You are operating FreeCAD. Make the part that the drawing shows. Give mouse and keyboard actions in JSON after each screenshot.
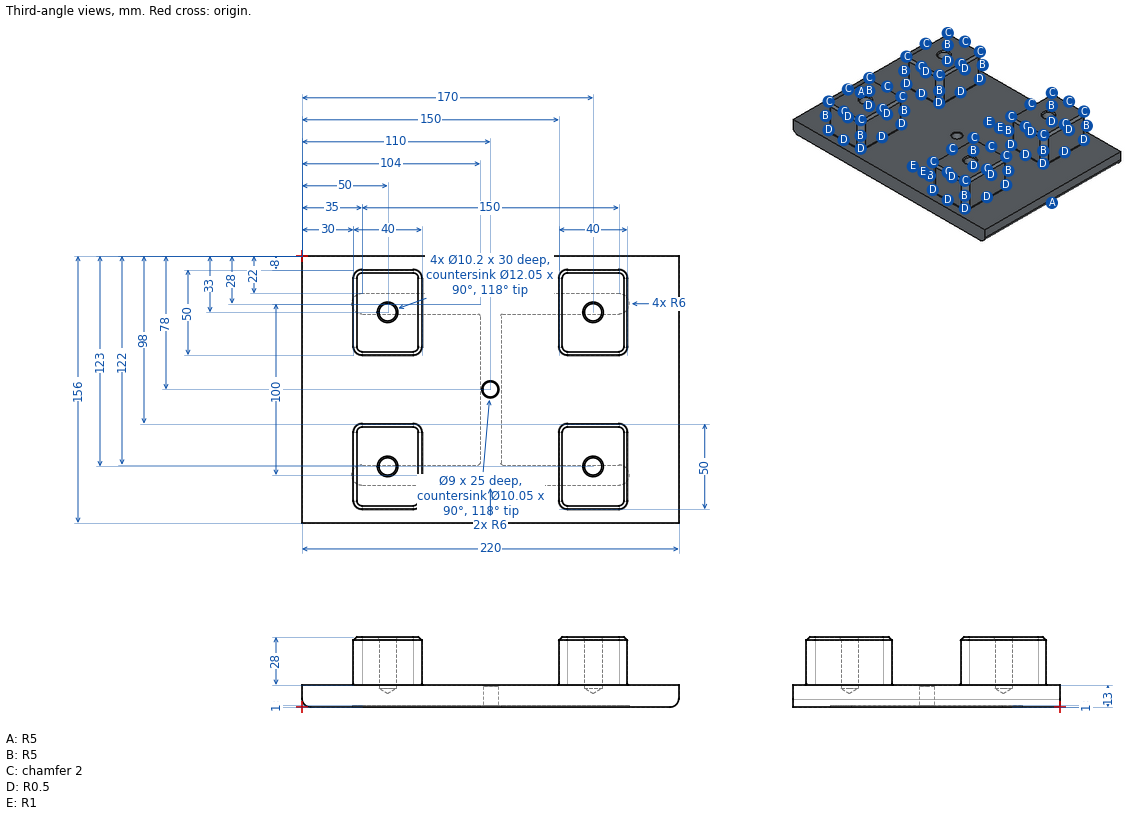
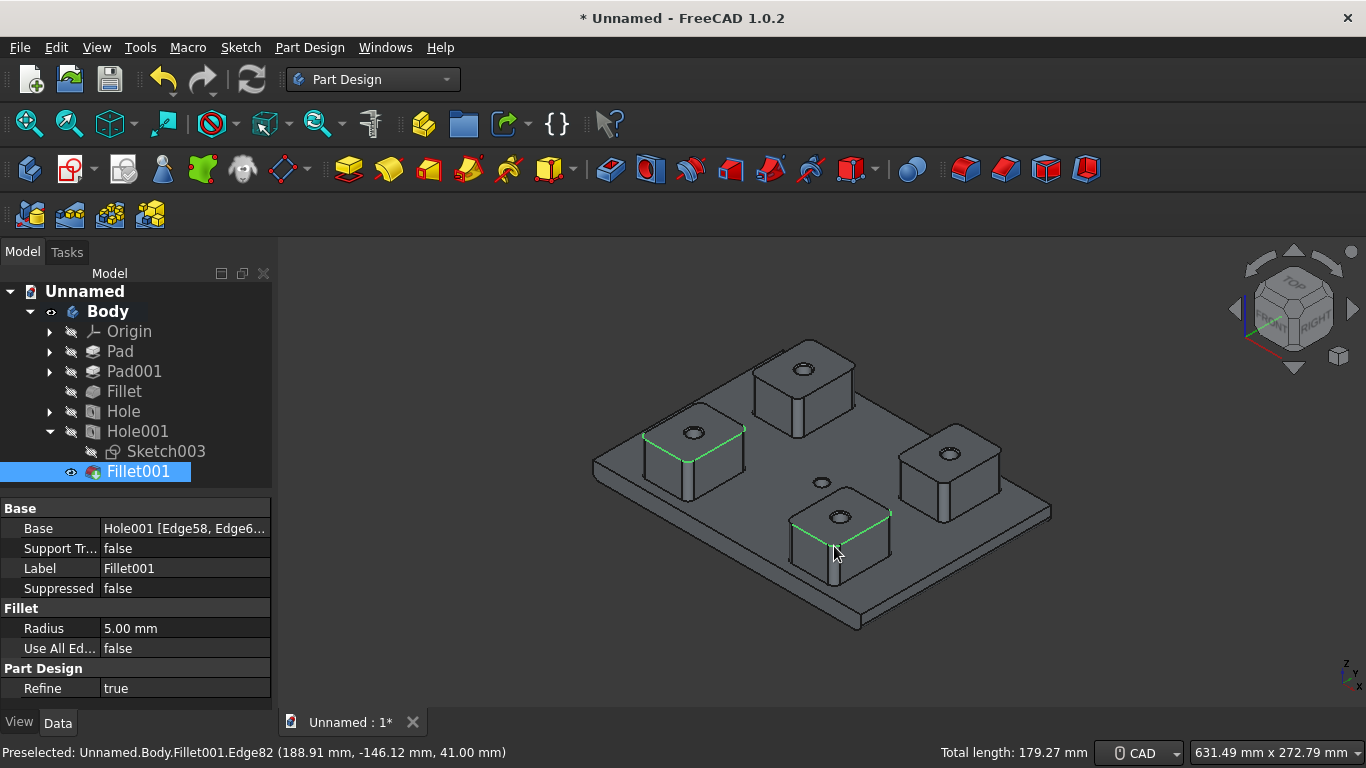
{"action": "left_click", "coordinate": [790, 517], "text": "ctrl"}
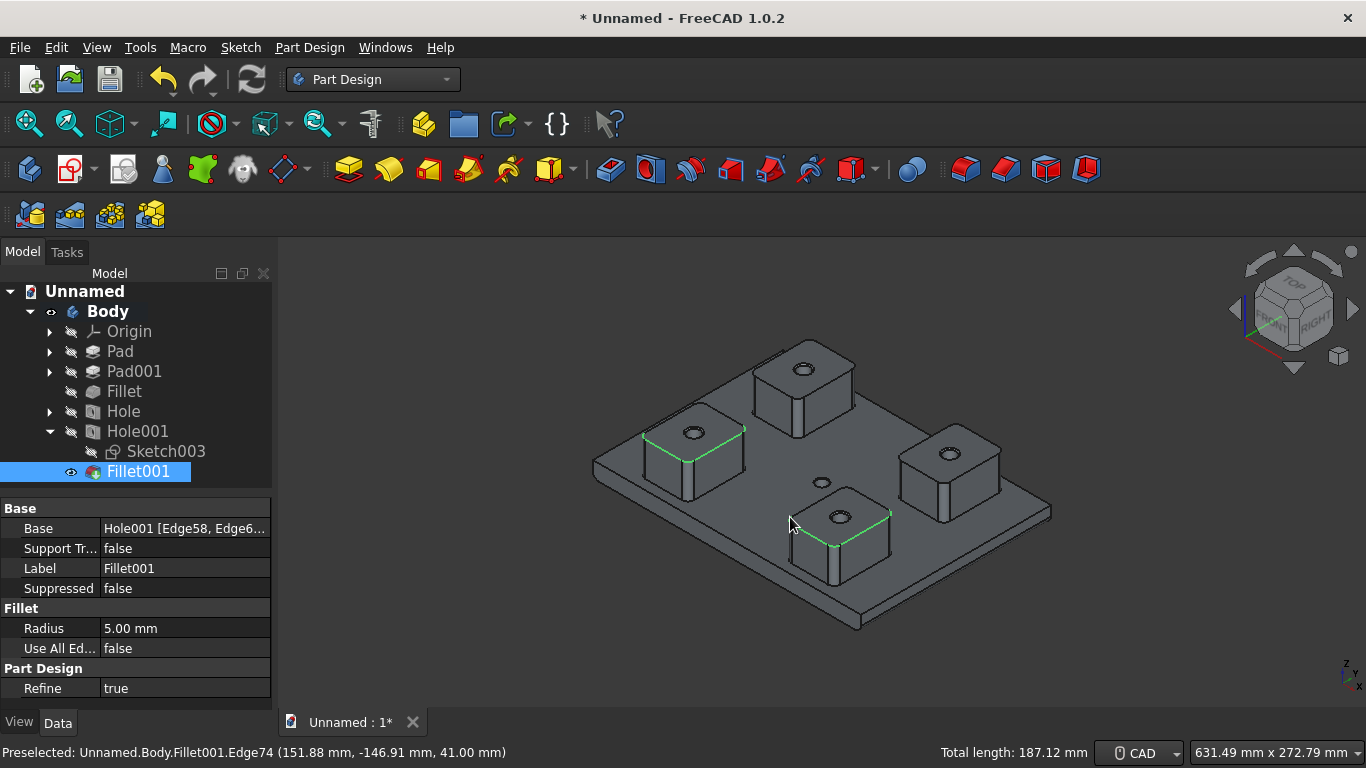
{"action": "left_click", "coordinate": [919, 470], "text": "ctrl"}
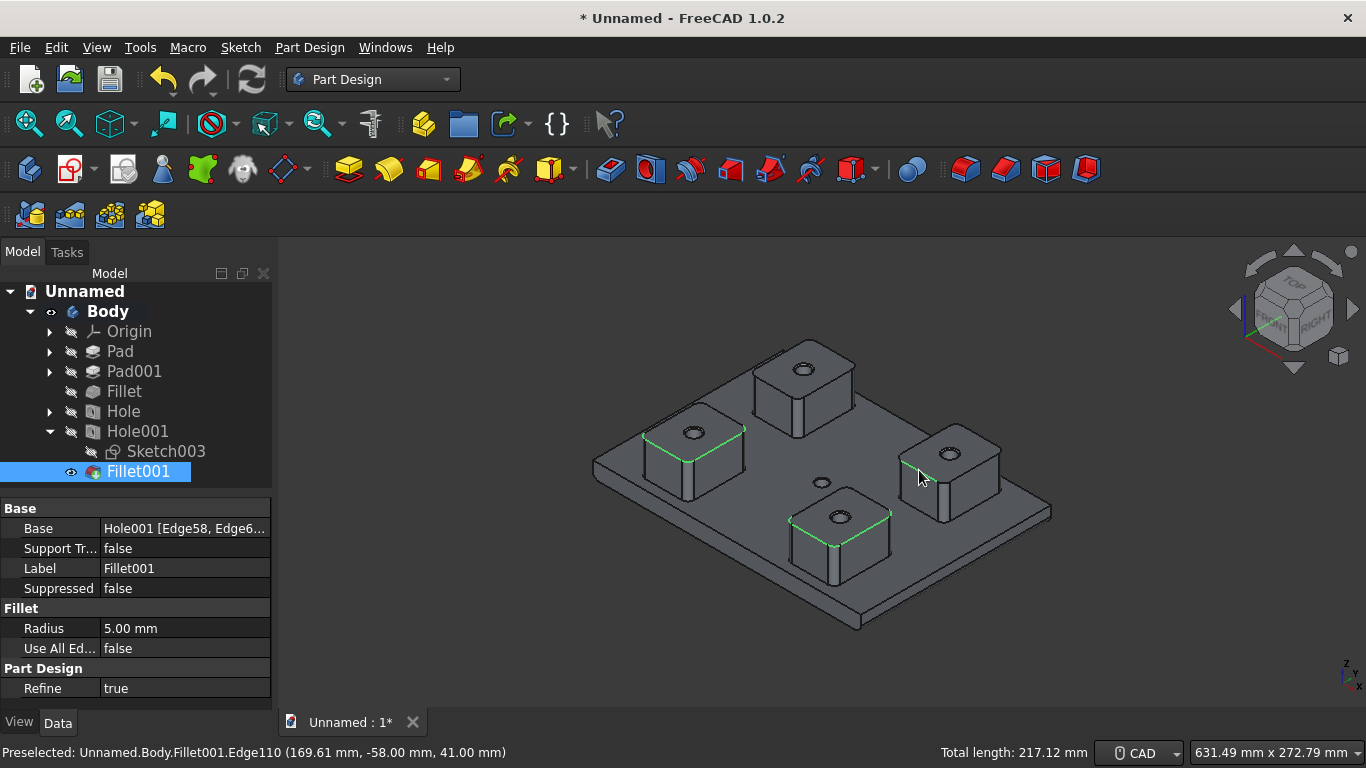
{"action": "left_click", "coordinate": [974, 467], "text": "ctrl"}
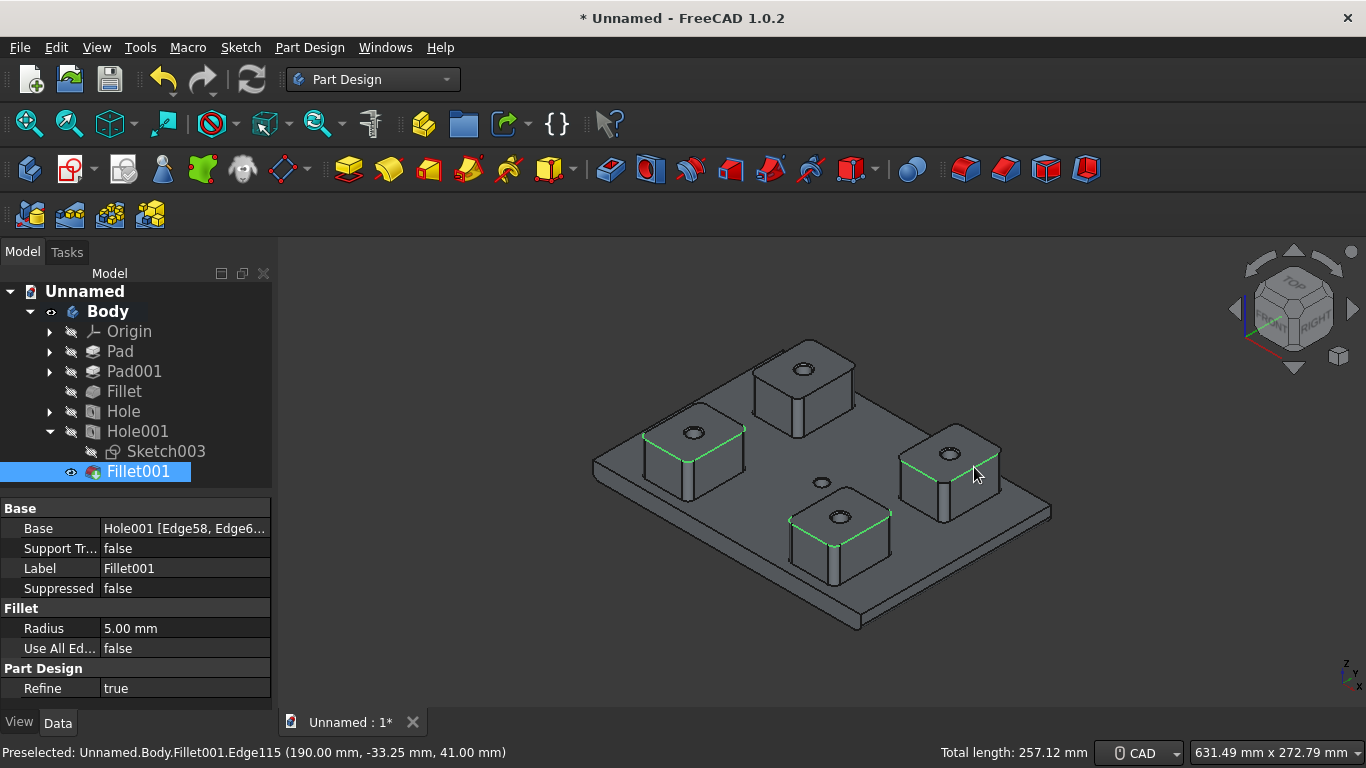
{"action": "left_click", "coordinate": [900, 453], "text": "ctrl"}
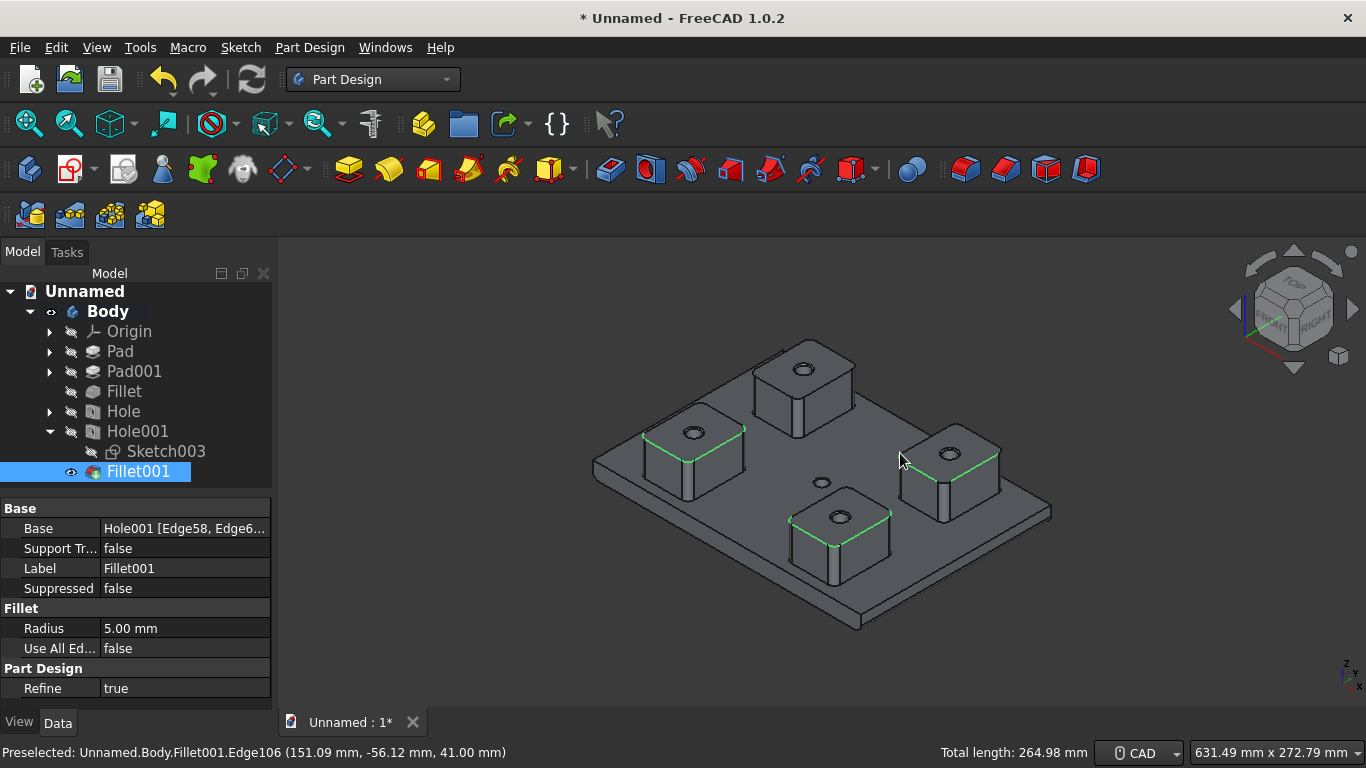
{"action": "left_click", "coordinate": [944, 482], "text": "ctrl"}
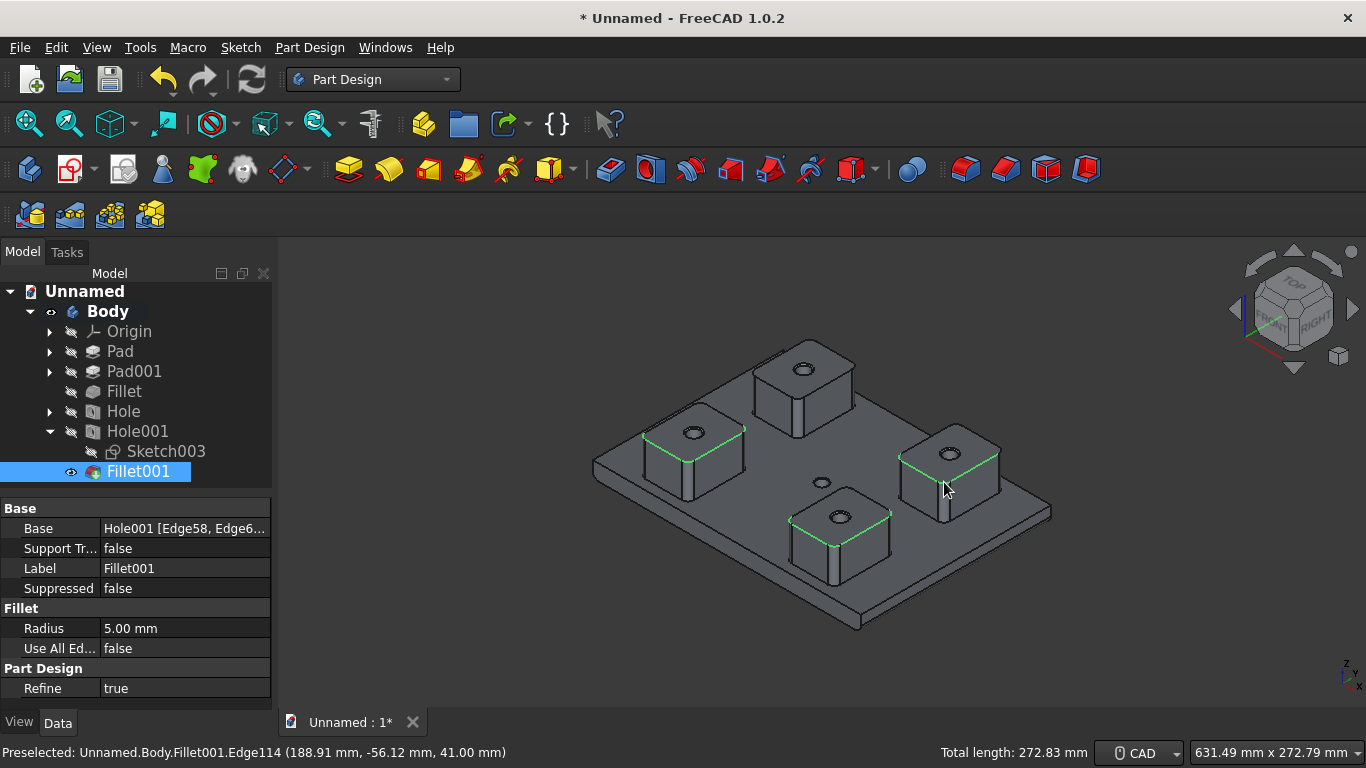
{"action": "left_click", "coordinate": [1000, 446], "text": "ctrl"}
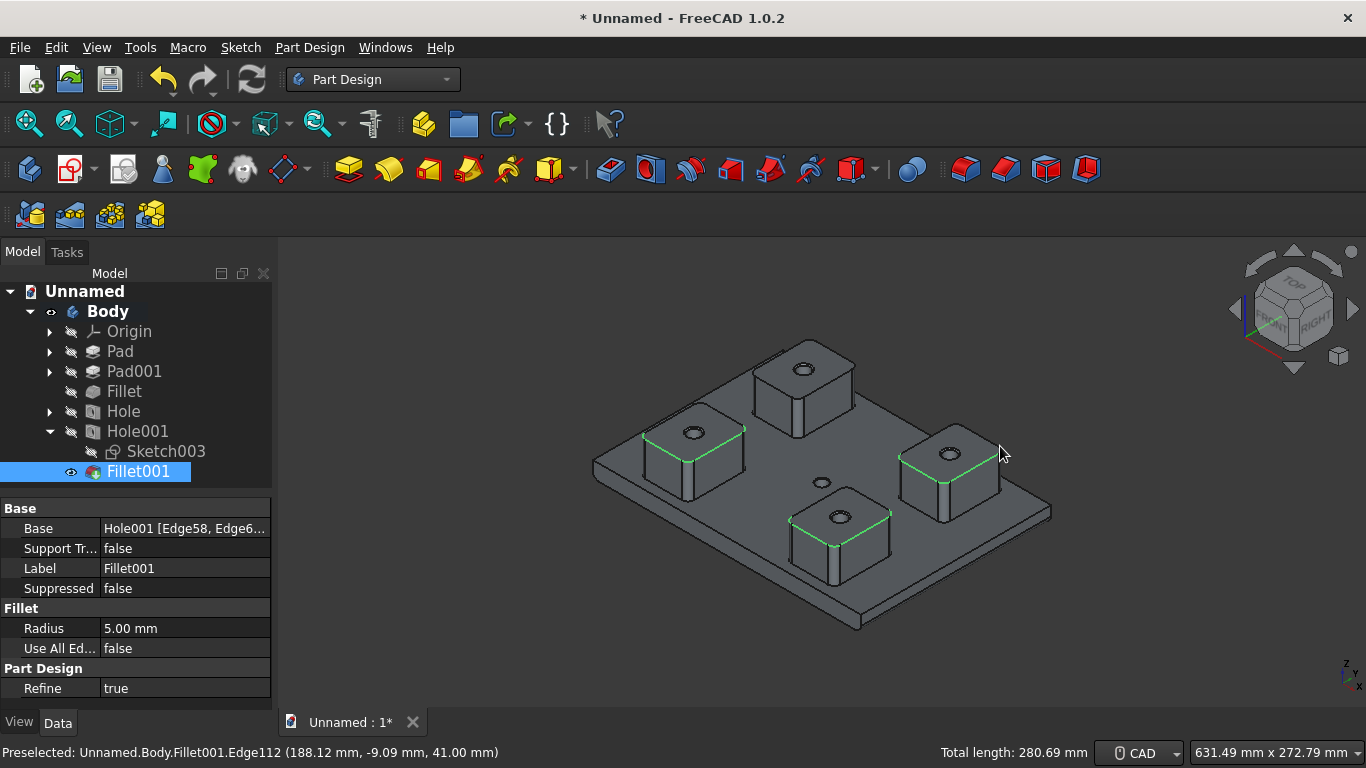
{"action": "left_click", "coordinate": [828, 382], "text": "ctrl"}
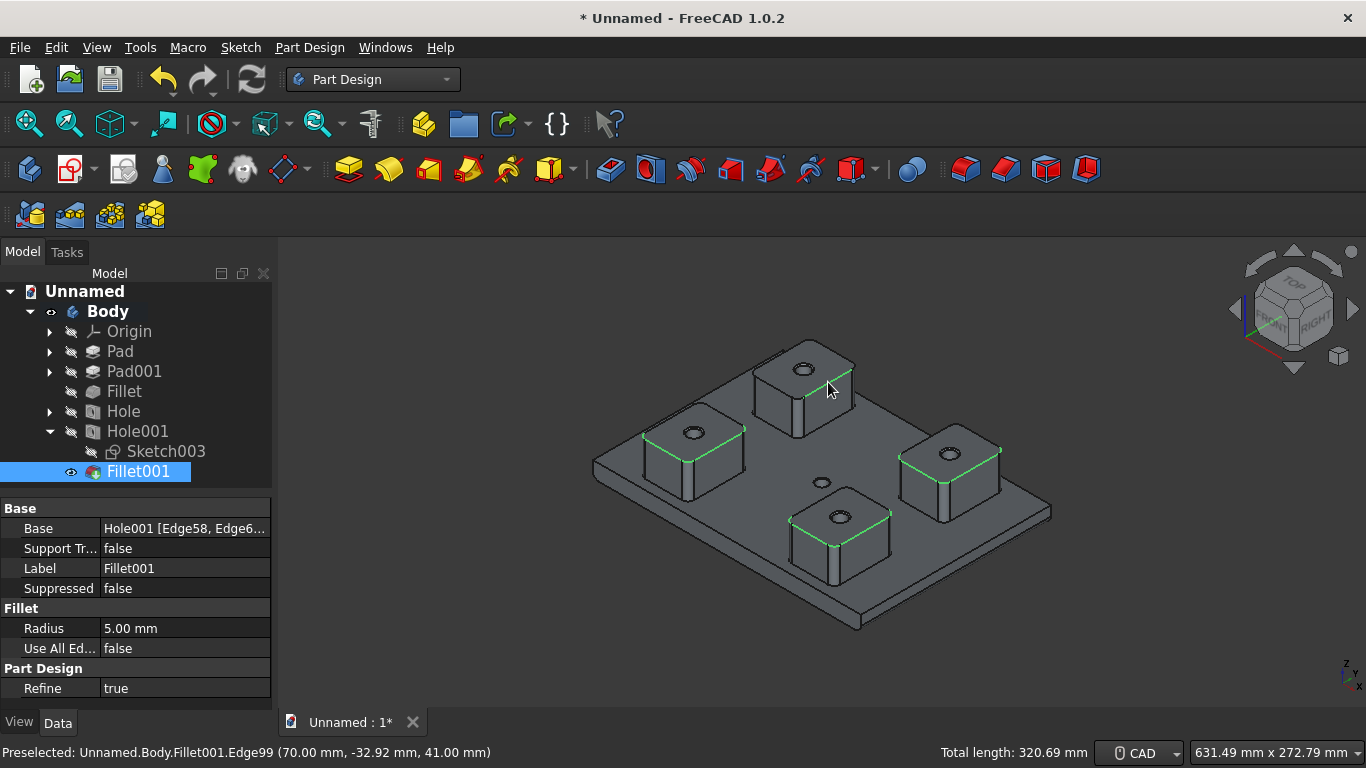
{"action": "left_click", "coordinate": [773, 386], "text": "ctrl"}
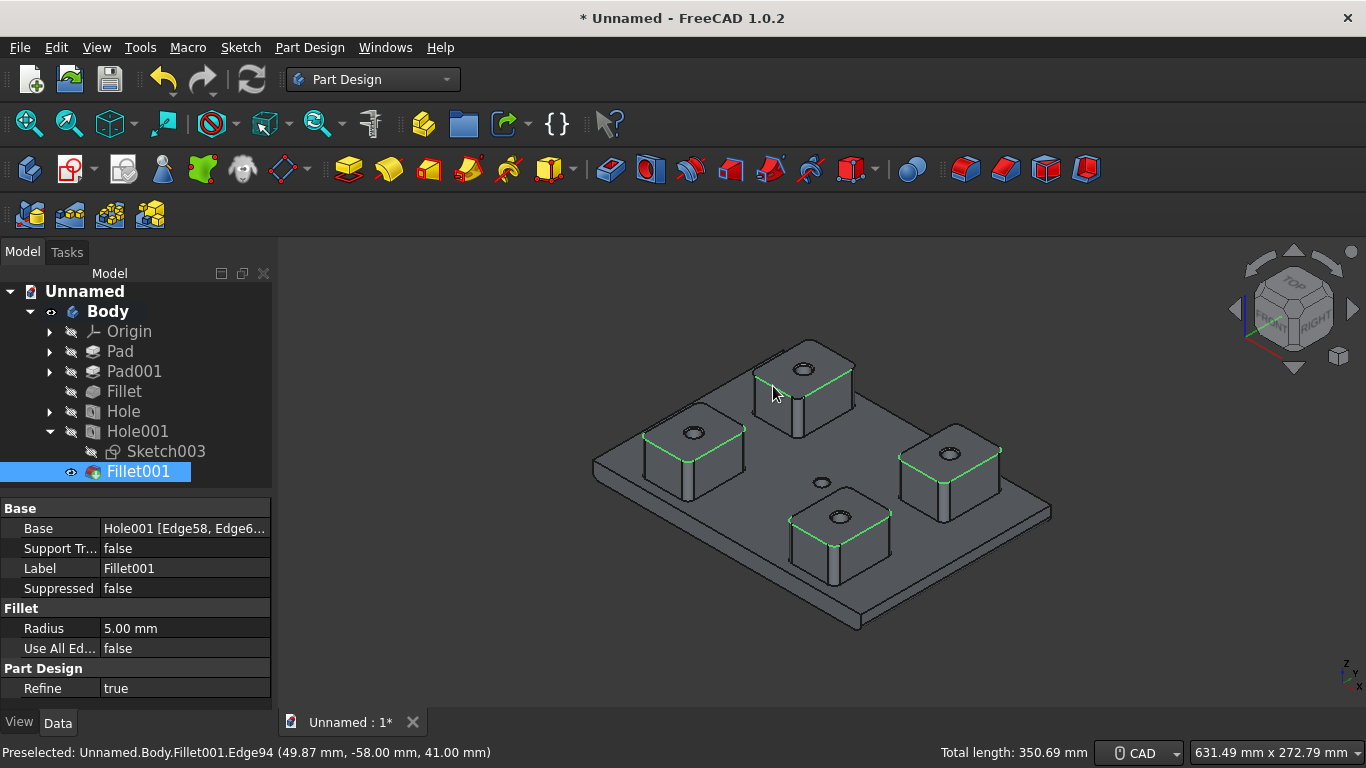
{"action": "left_click", "coordinate": [853, 362], "text": "ctrl"}